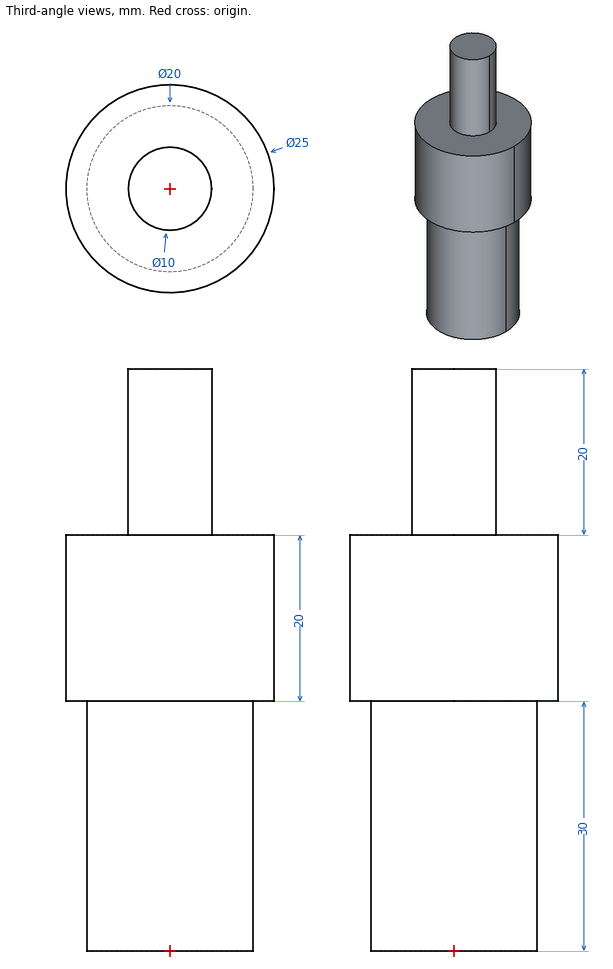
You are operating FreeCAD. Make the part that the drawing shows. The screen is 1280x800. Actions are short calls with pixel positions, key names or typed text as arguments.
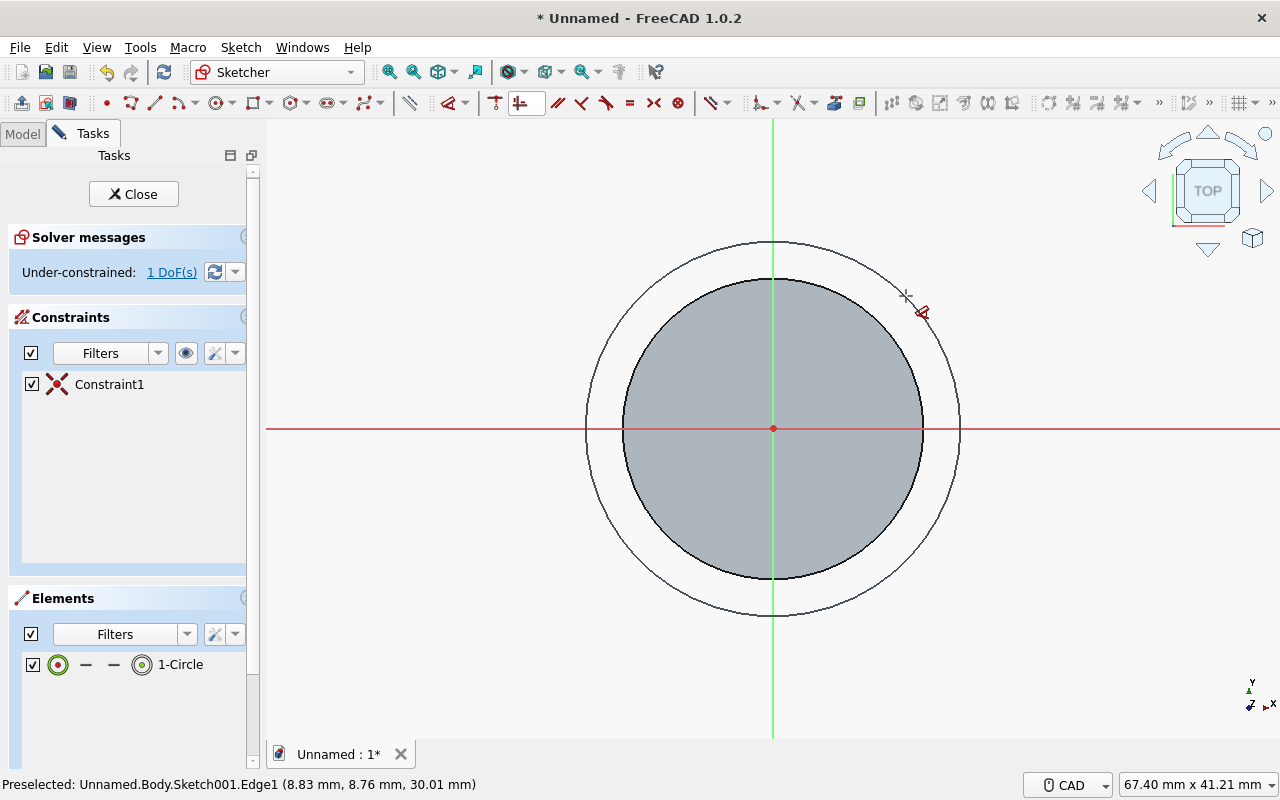
click(905, 296)
click(928, 273)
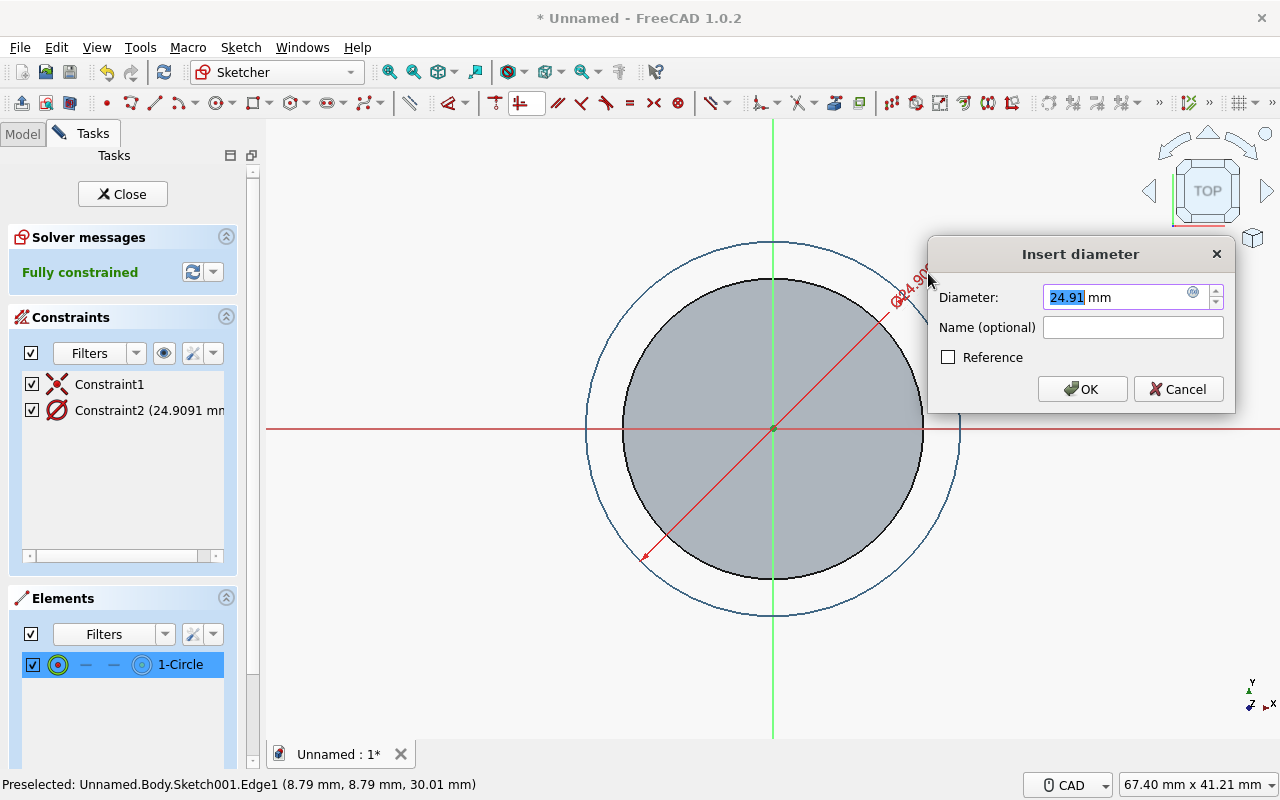
text(25)
key(Return)
key(Escape)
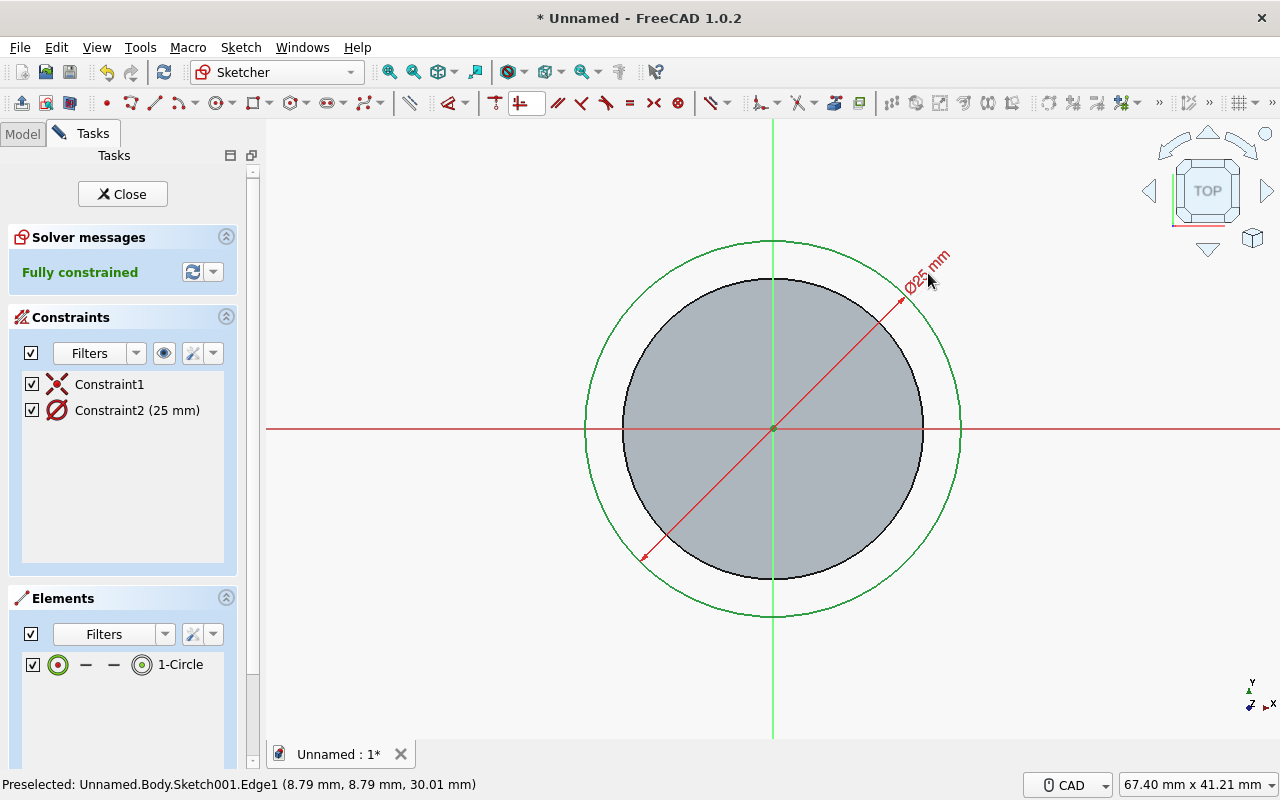
click(123, 194)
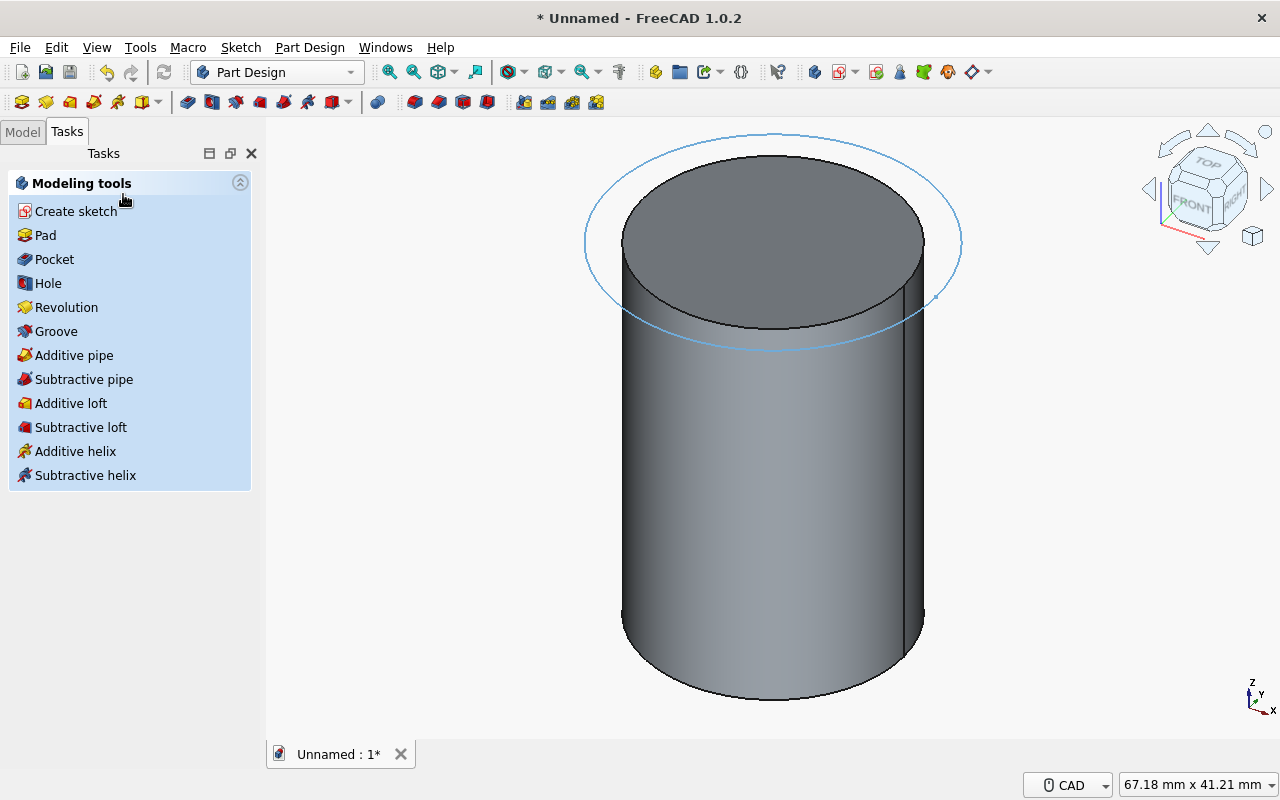
click(22, 102)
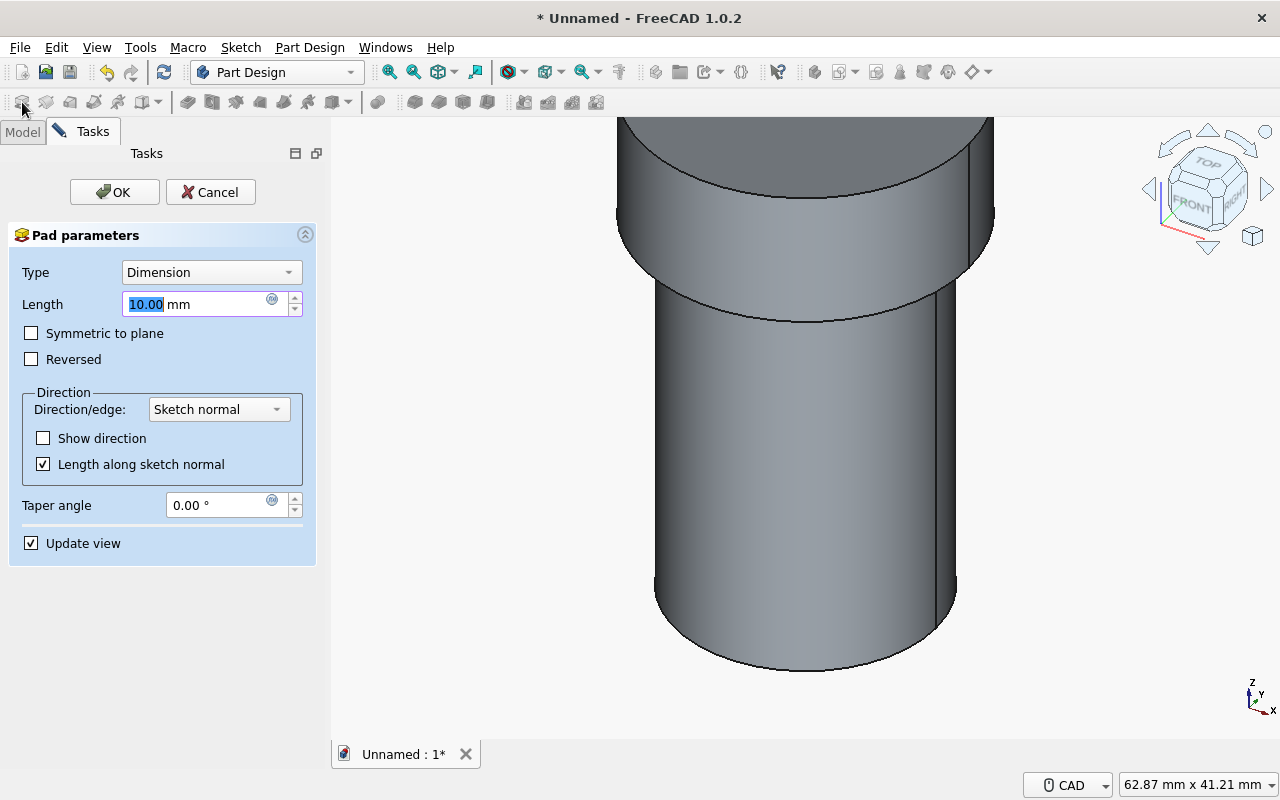
text(20)
key(Tab)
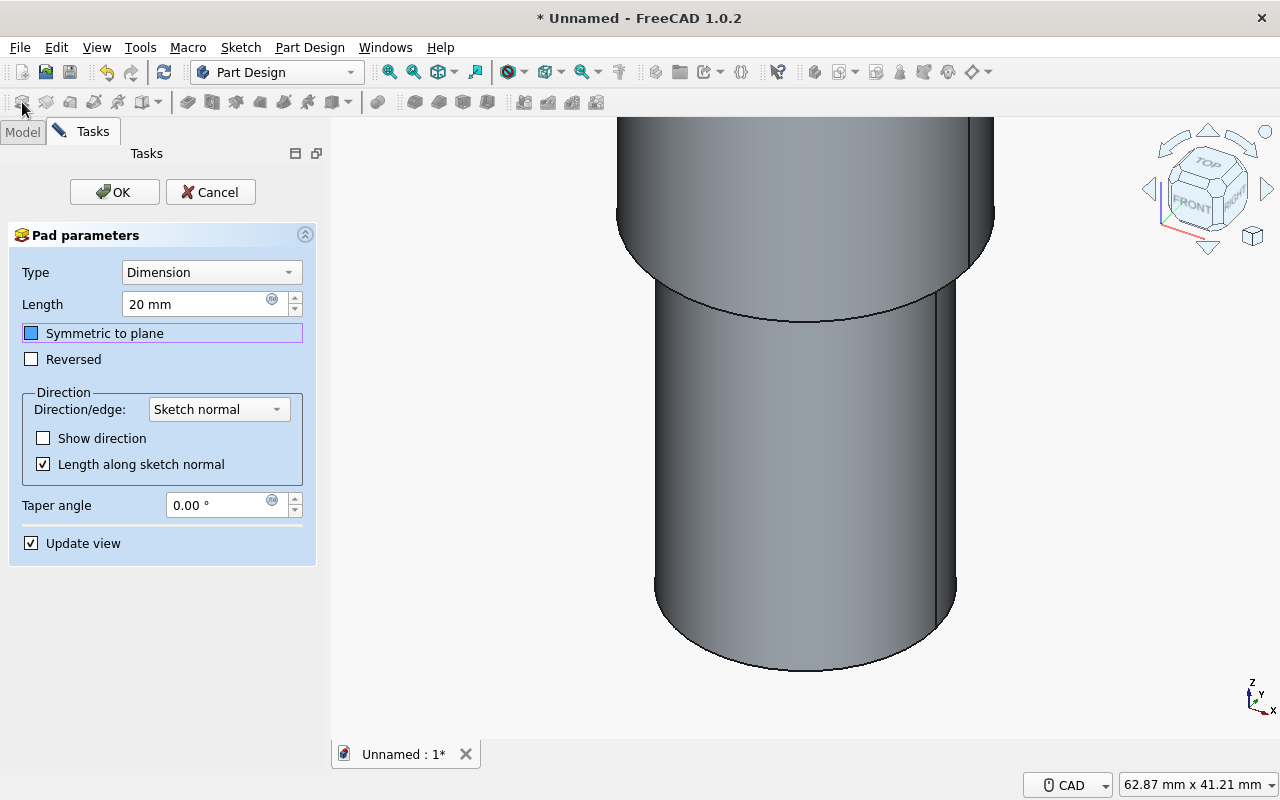
click(115, 192)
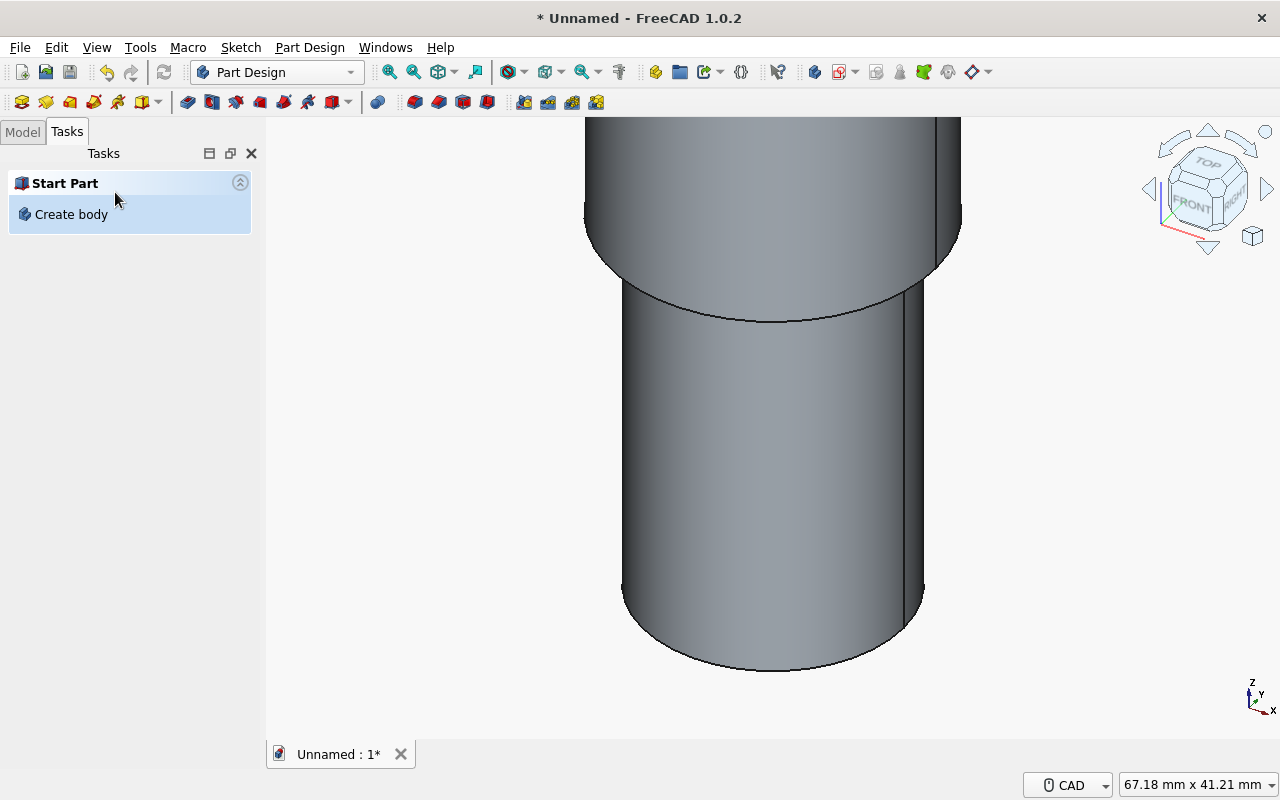
key(v)
key(f)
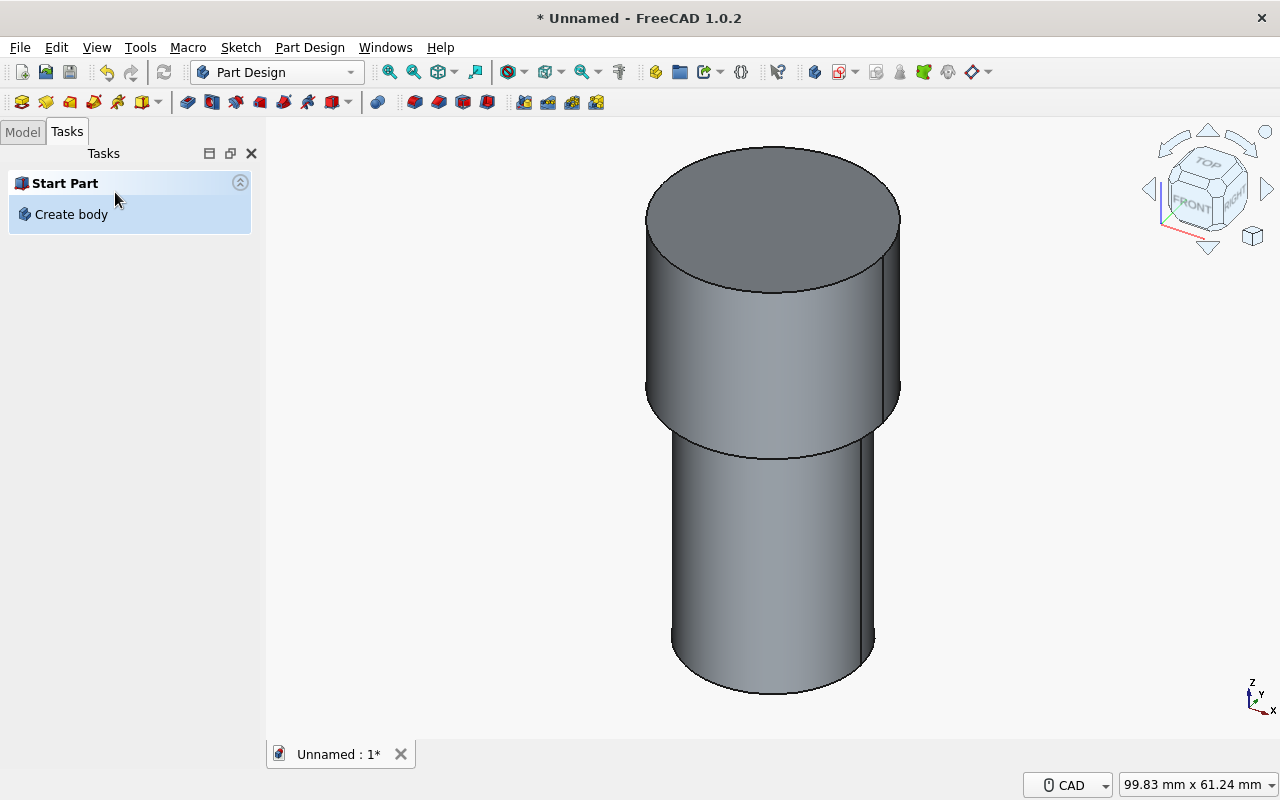
click(773, 219)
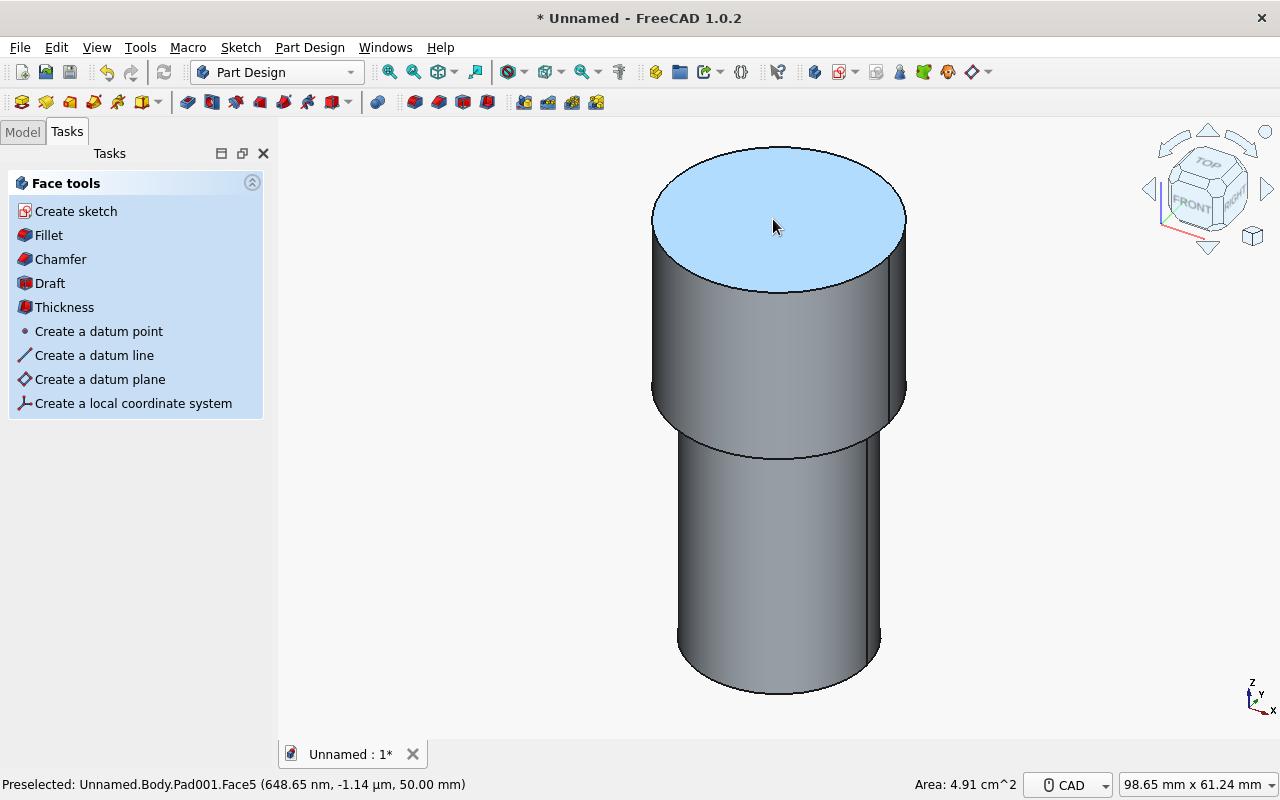
click(840, 72)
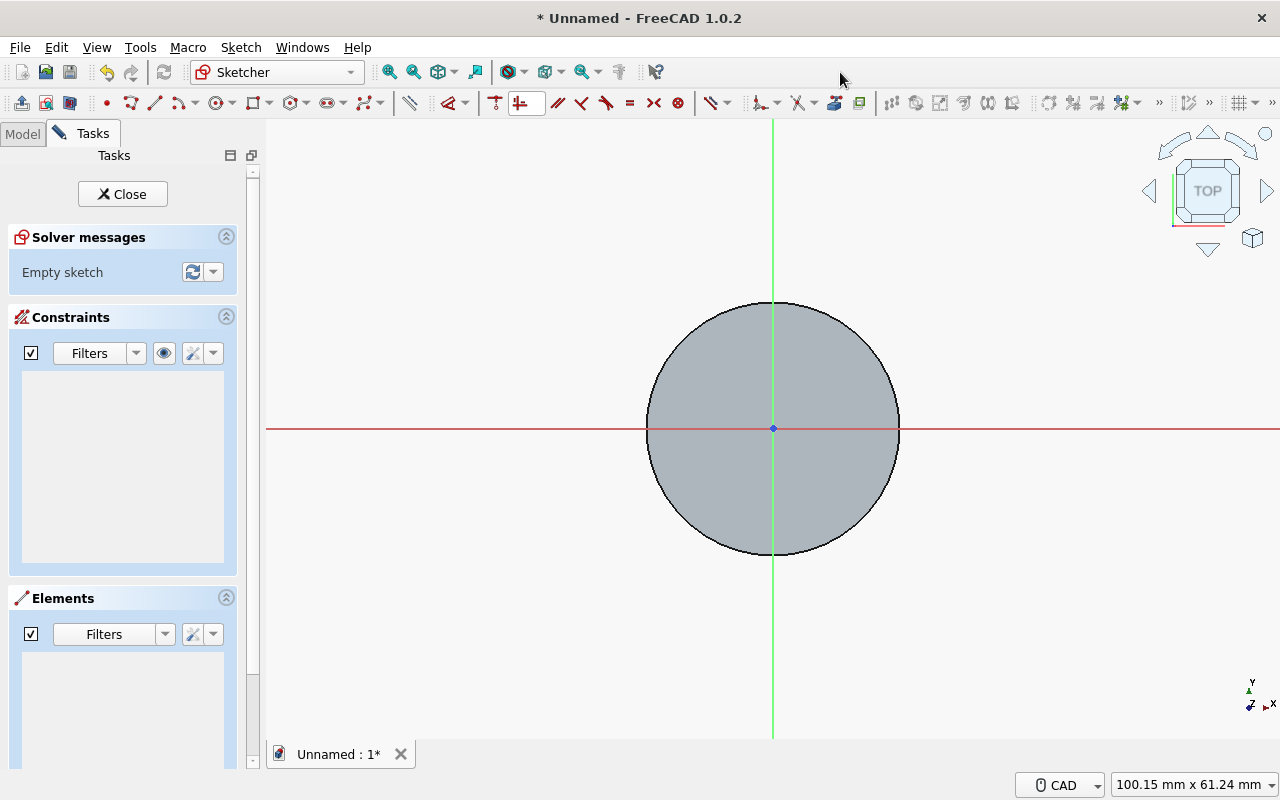
scroll(795, 429, up, 7)